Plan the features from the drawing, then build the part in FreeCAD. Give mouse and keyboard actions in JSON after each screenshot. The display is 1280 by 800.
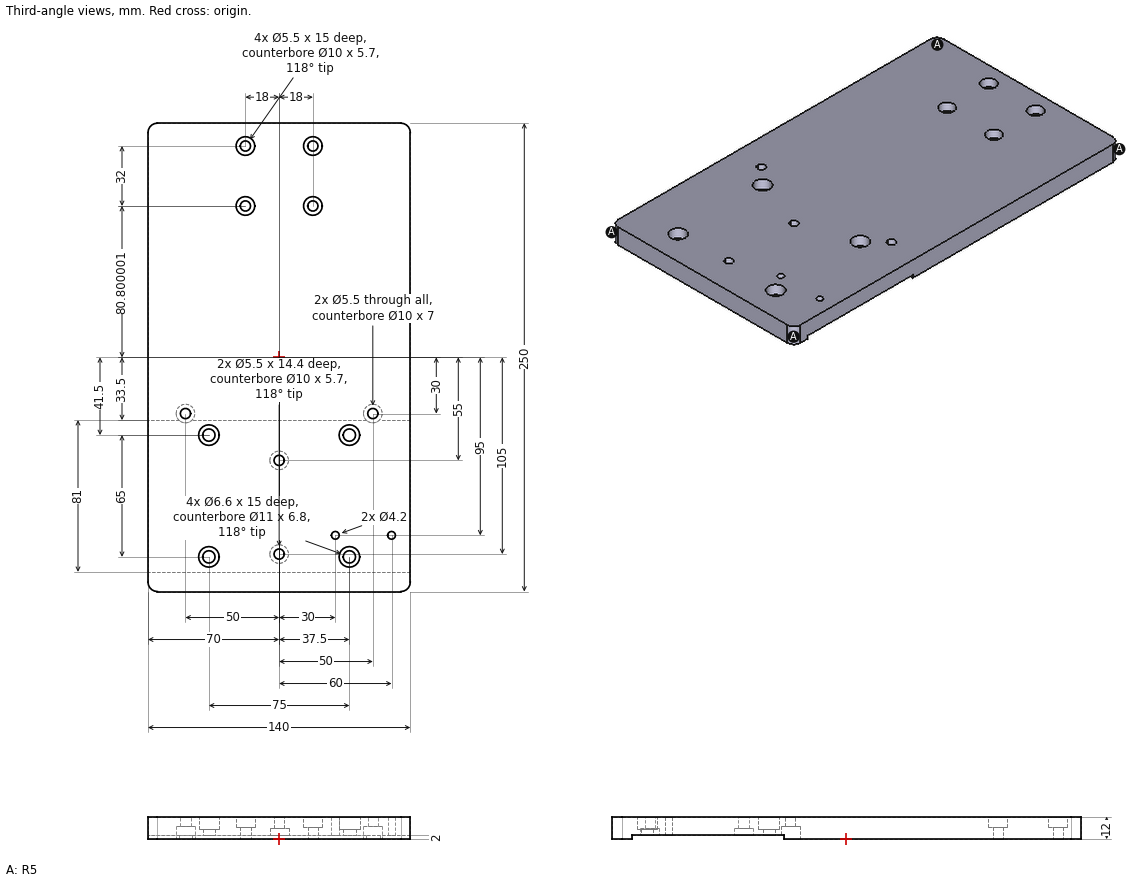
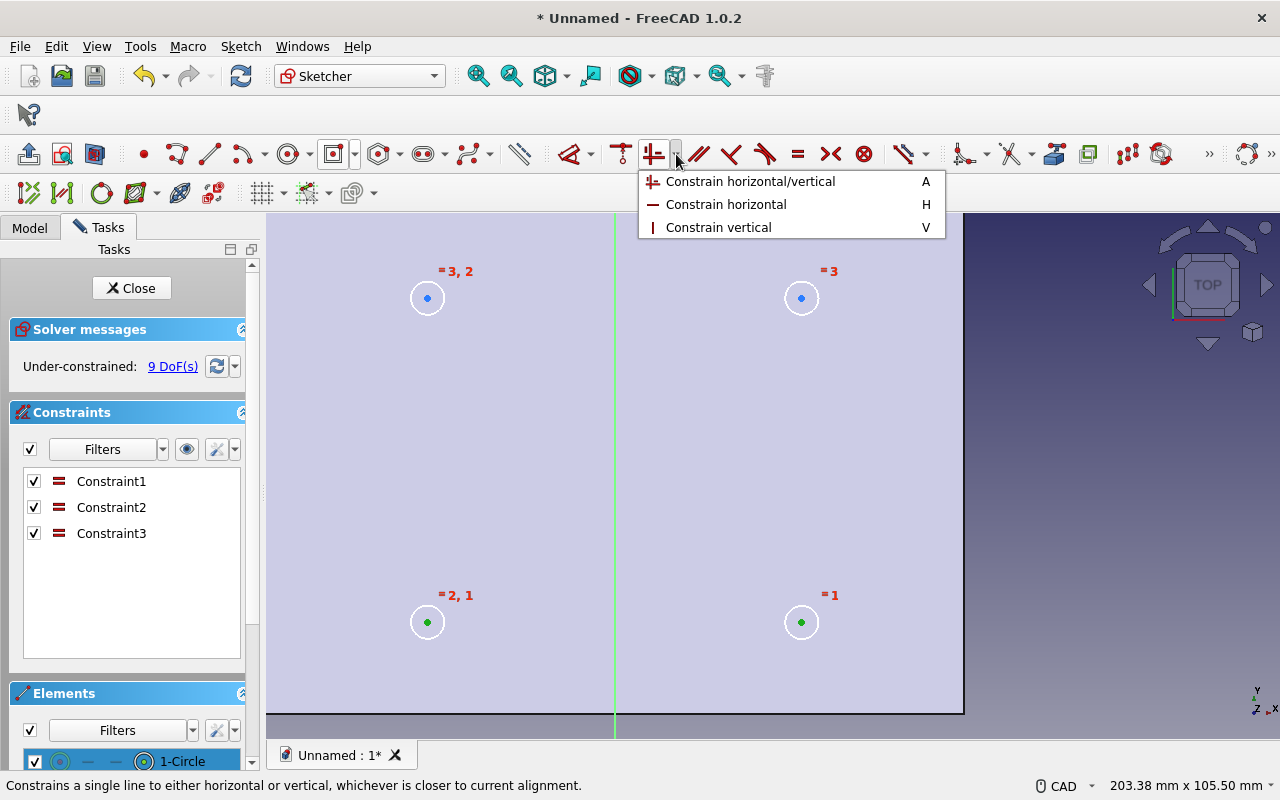
{"action": "left_click", "coordinate": [792, 204]}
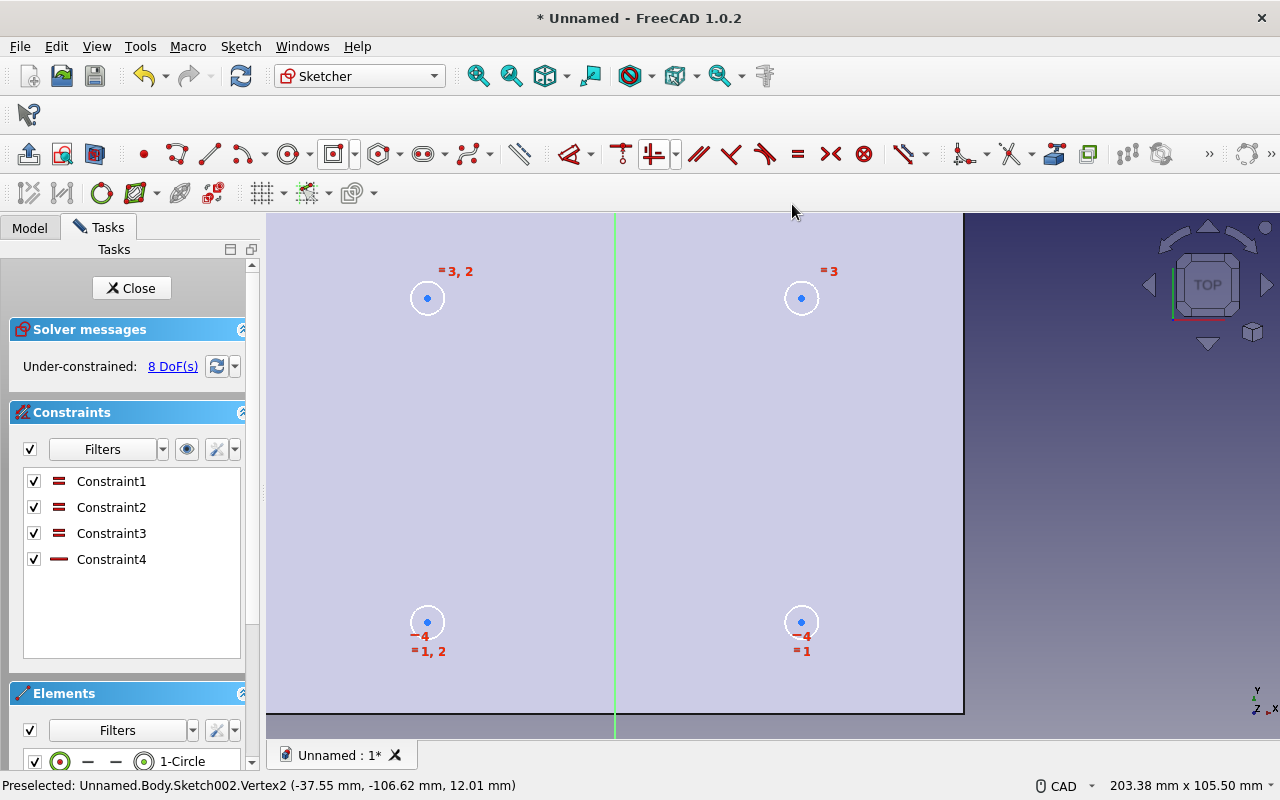
{"action": "left_click", "coordinate": [428, 623]}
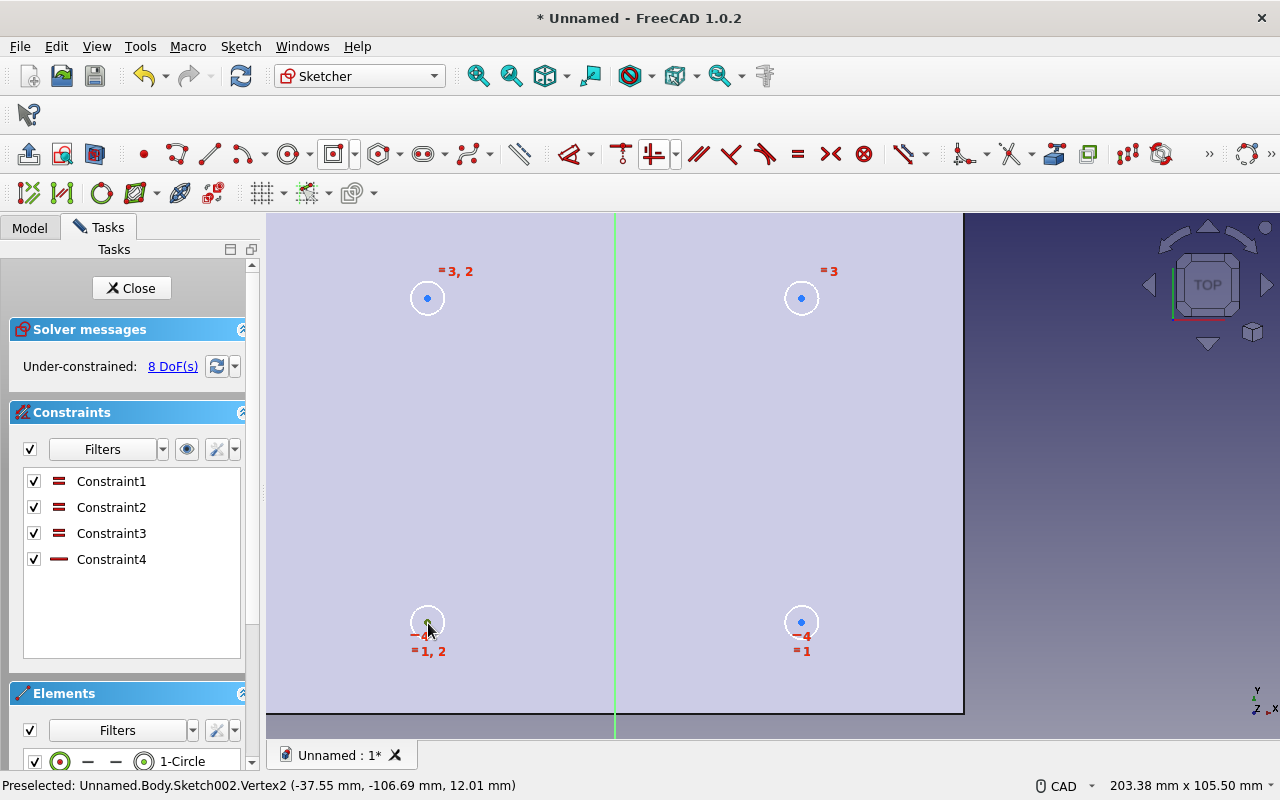
{"action": "left_click", "coordinate": [428, 298]}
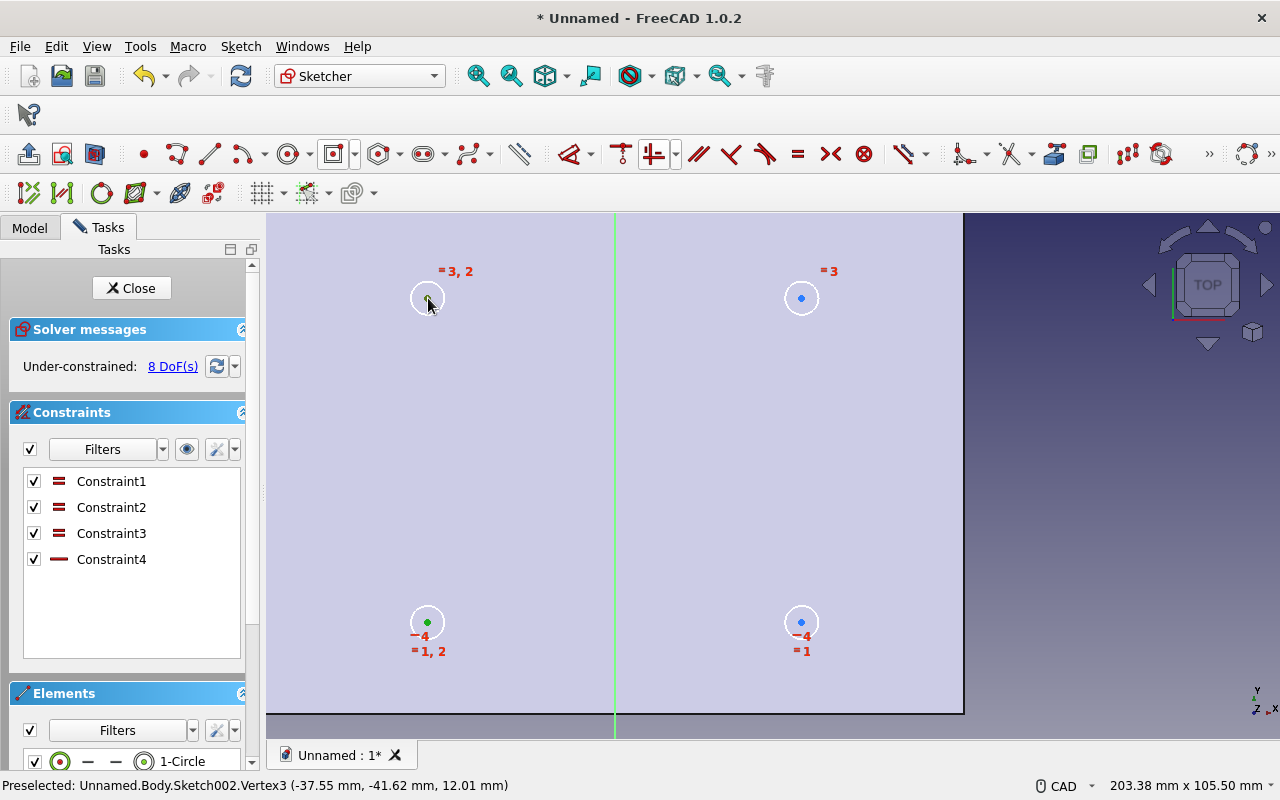
{"action": "left_click", "coordinate": [676, 154]}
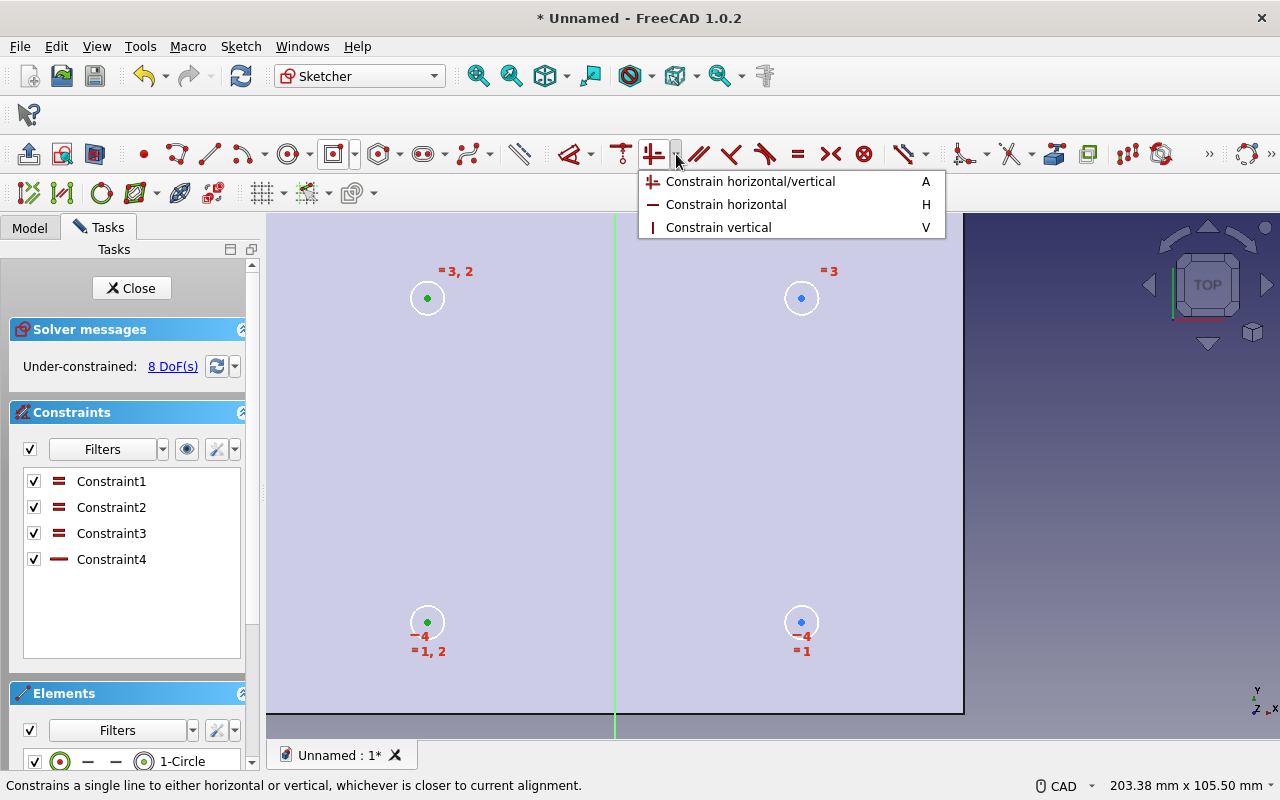
{"action": "left_click", "coordinate": [792, 228]}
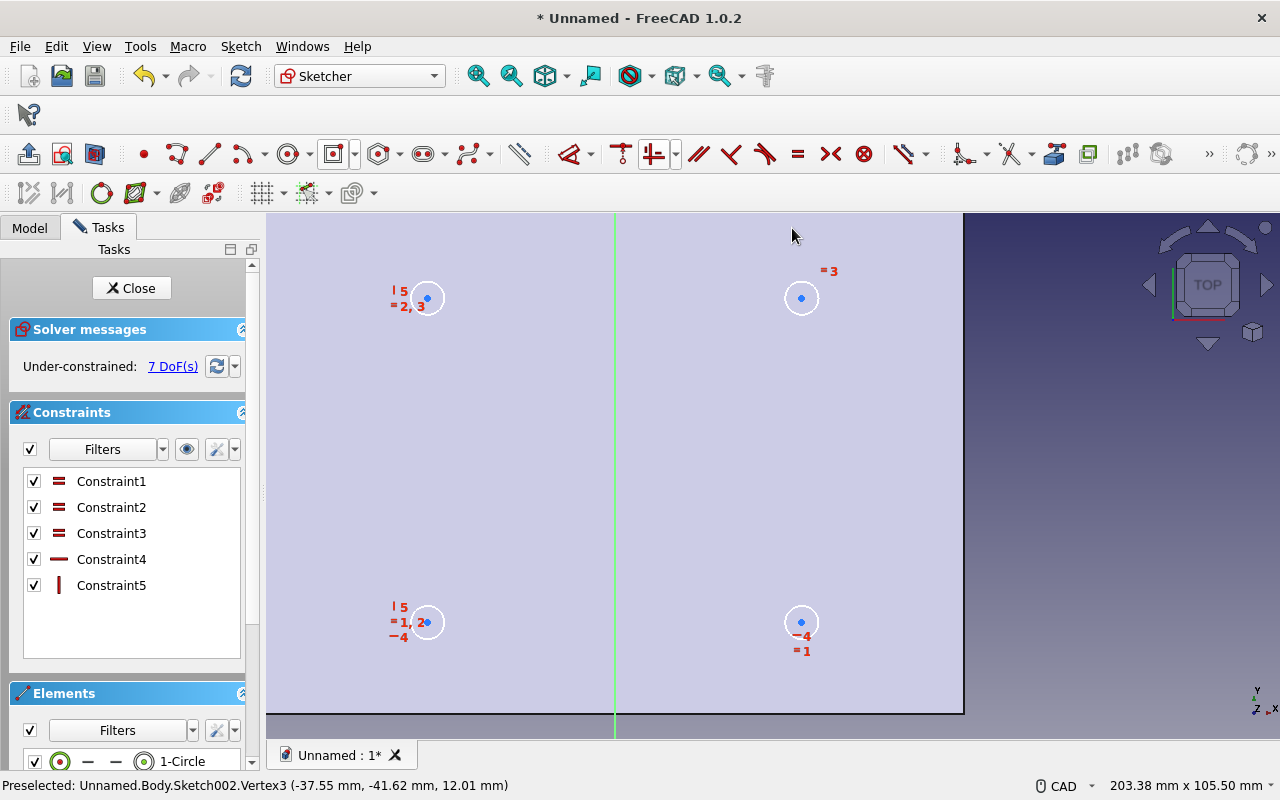
{"action": "left_click", "coordinate": [802, 623]}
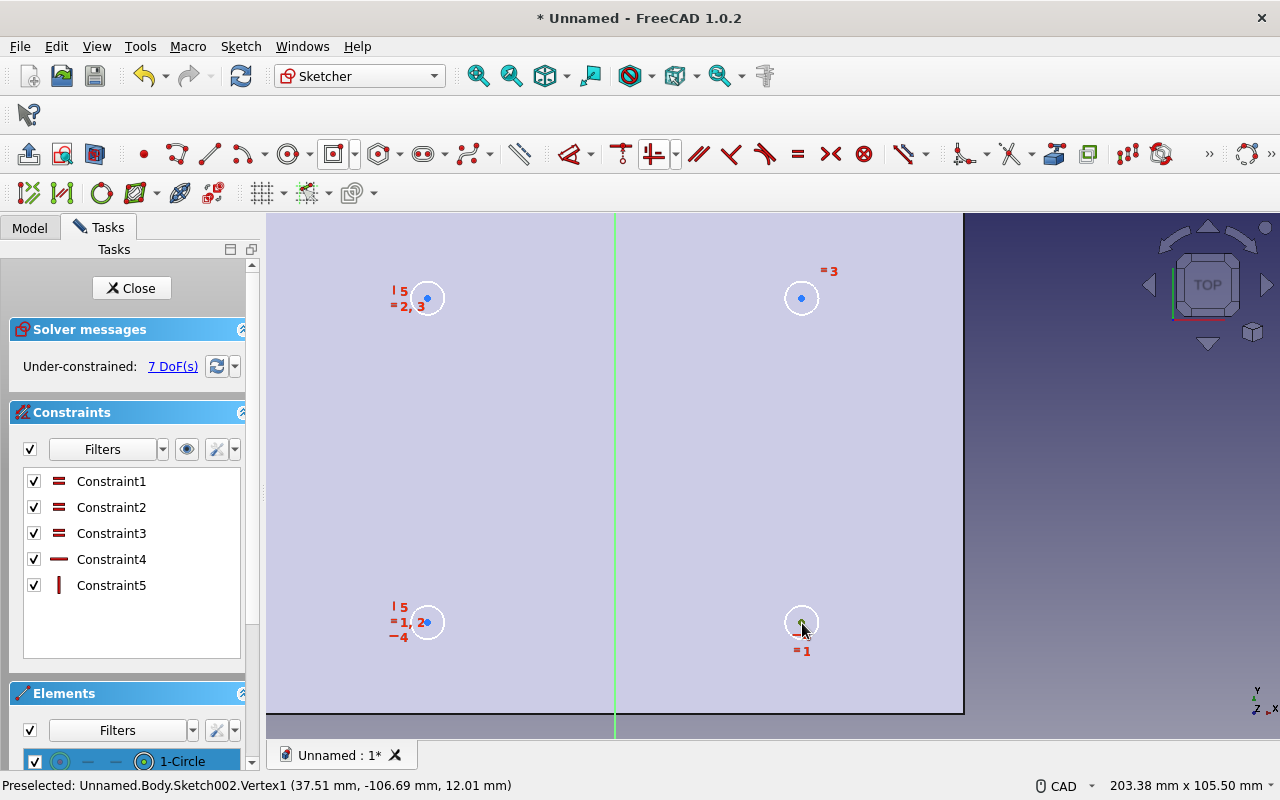
{"action": "left_click", "coordinate": [802, 298]}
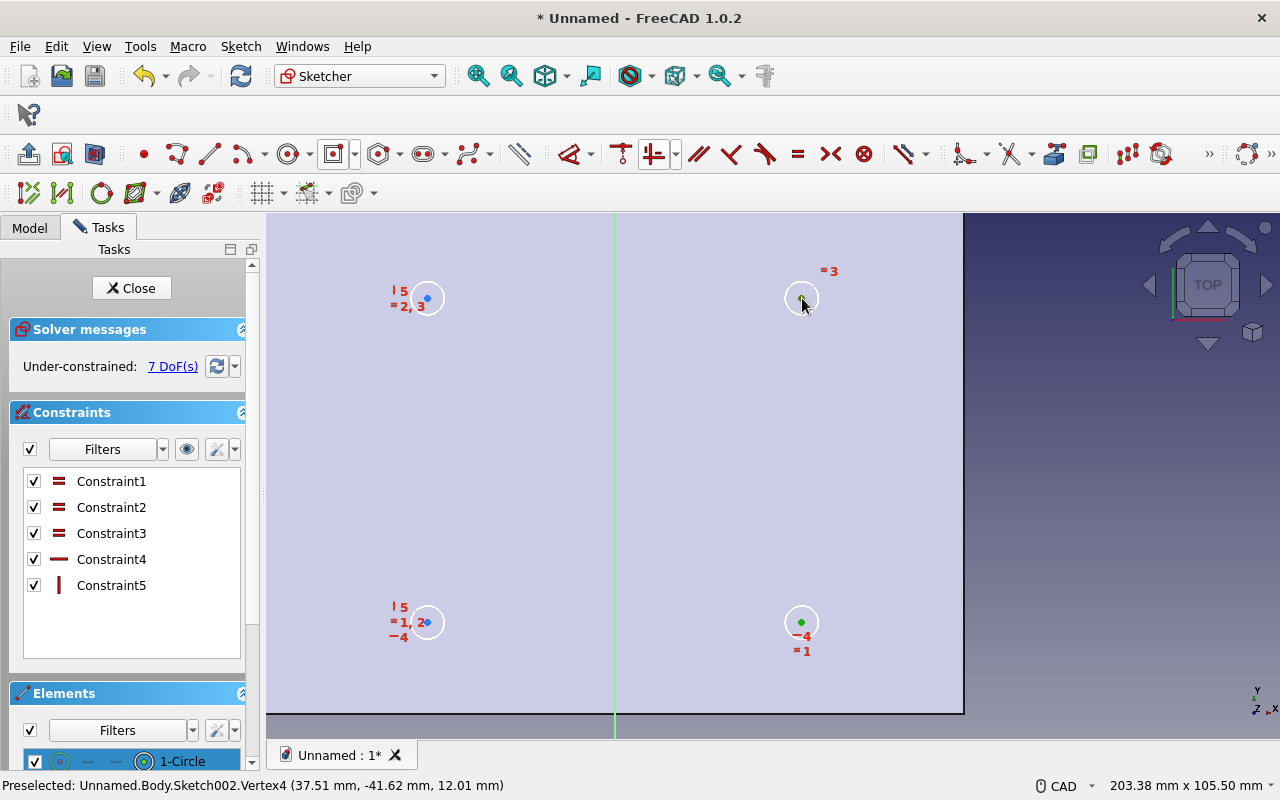
{"action": "left_click", "coordinate": [676, 154]}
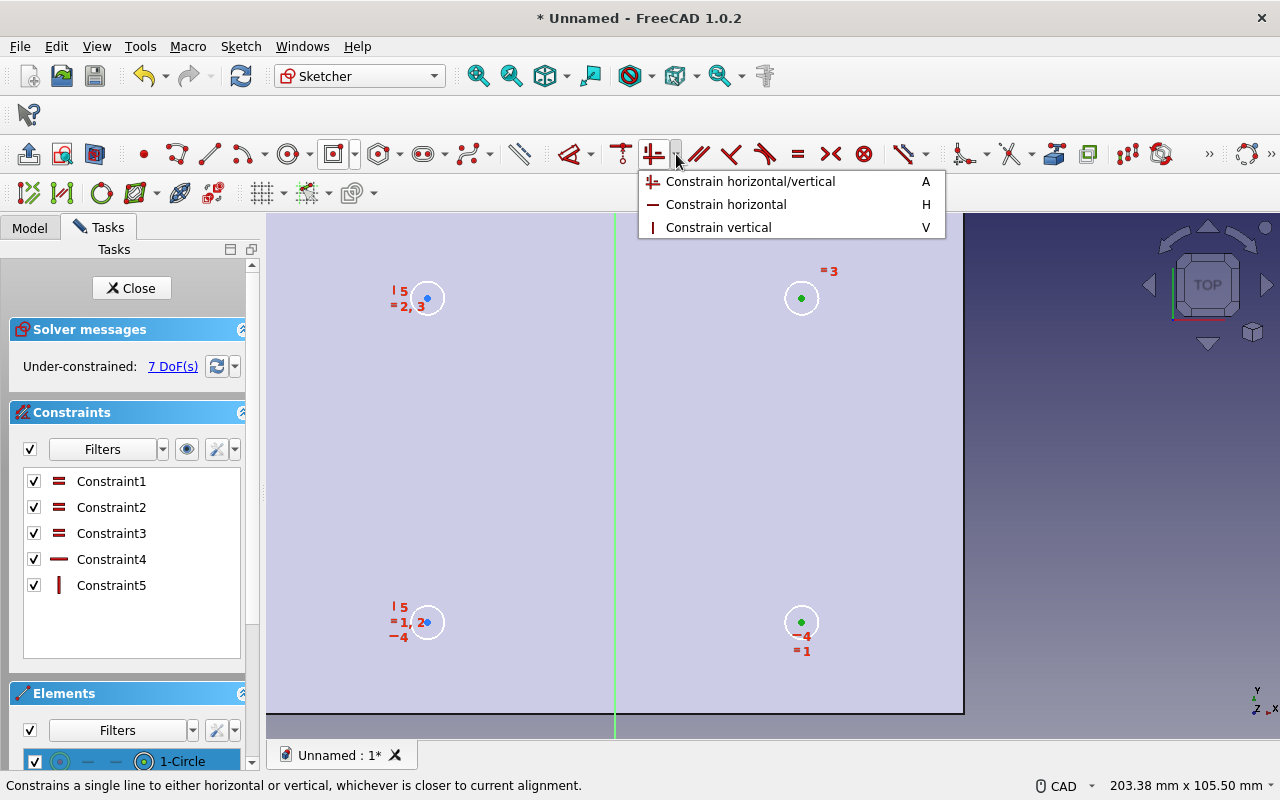
{"action": "left_click", "coordinate": [792, 228]}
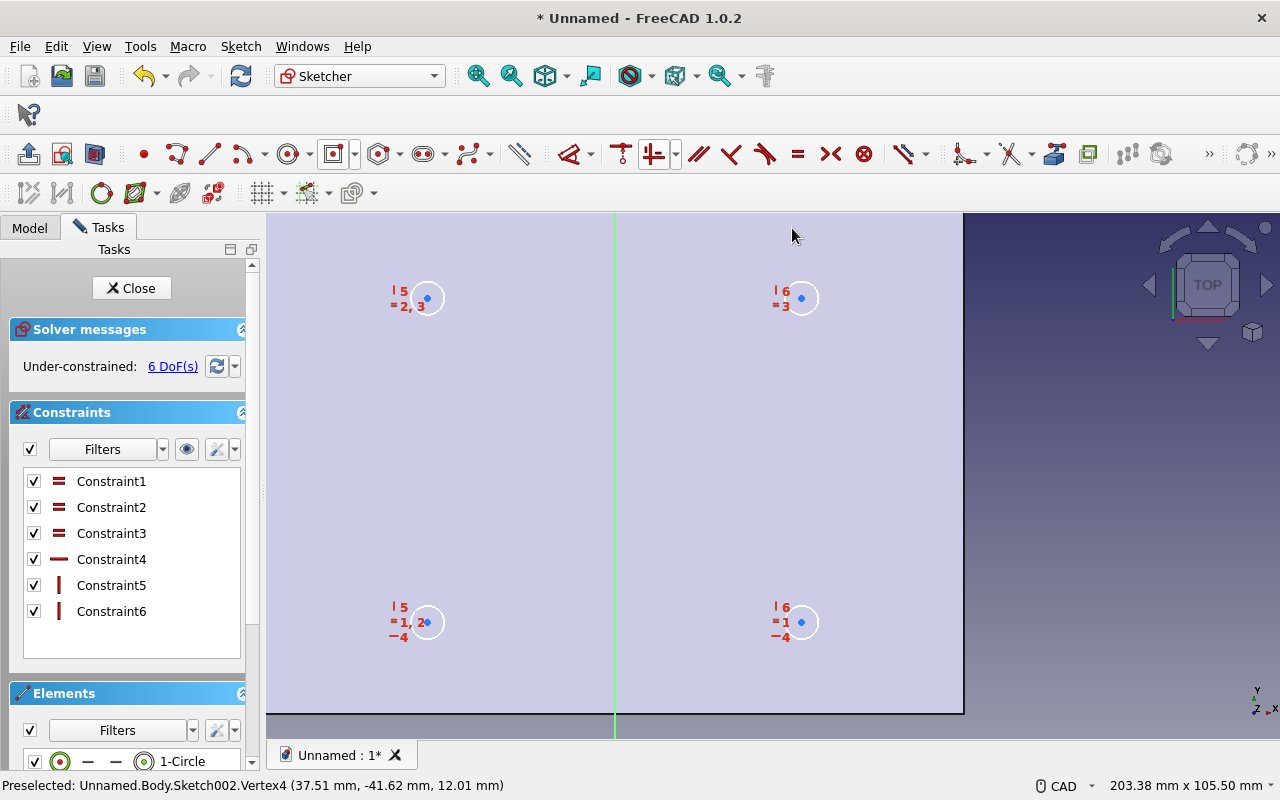
{"action": "left_click", "coordinate": [428, 298]}